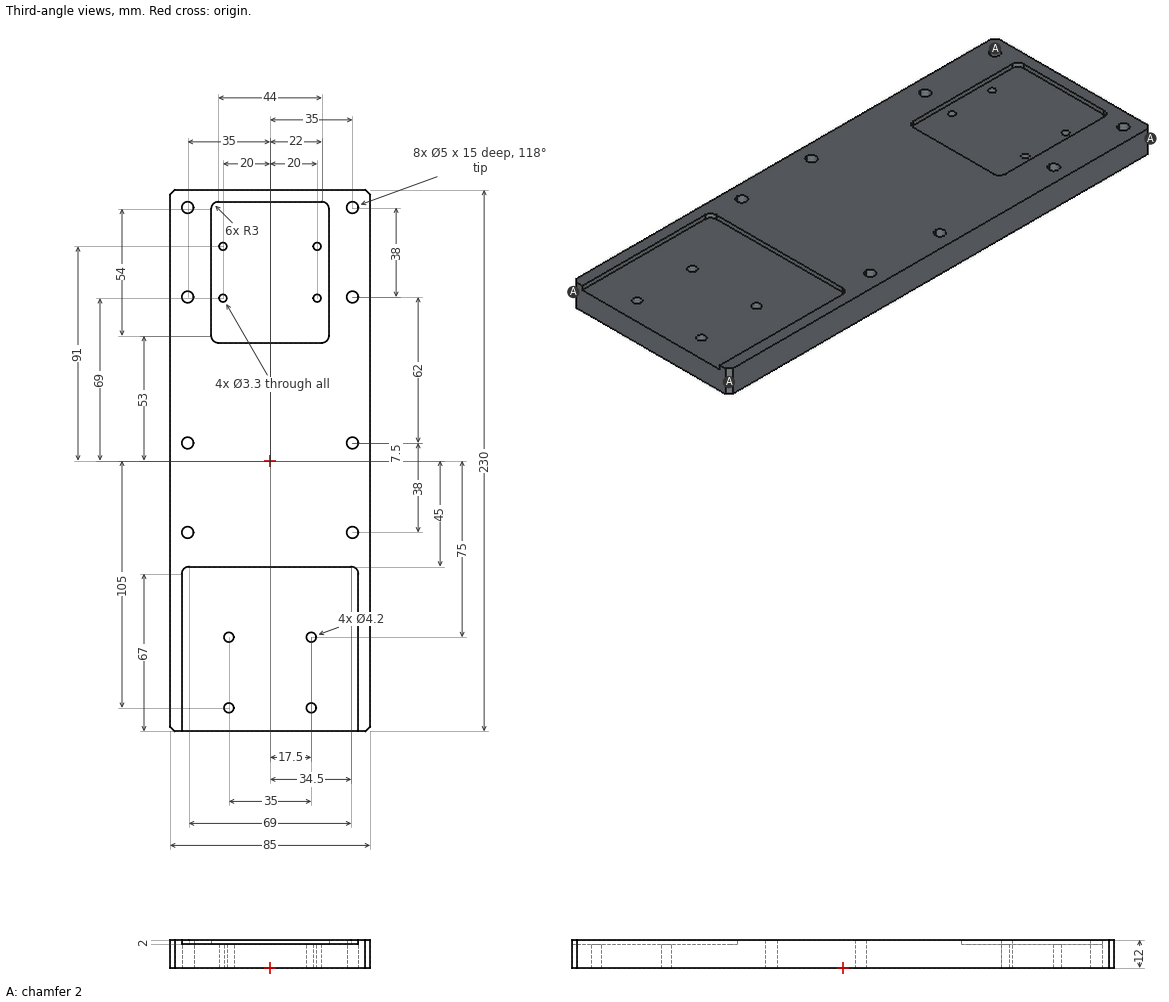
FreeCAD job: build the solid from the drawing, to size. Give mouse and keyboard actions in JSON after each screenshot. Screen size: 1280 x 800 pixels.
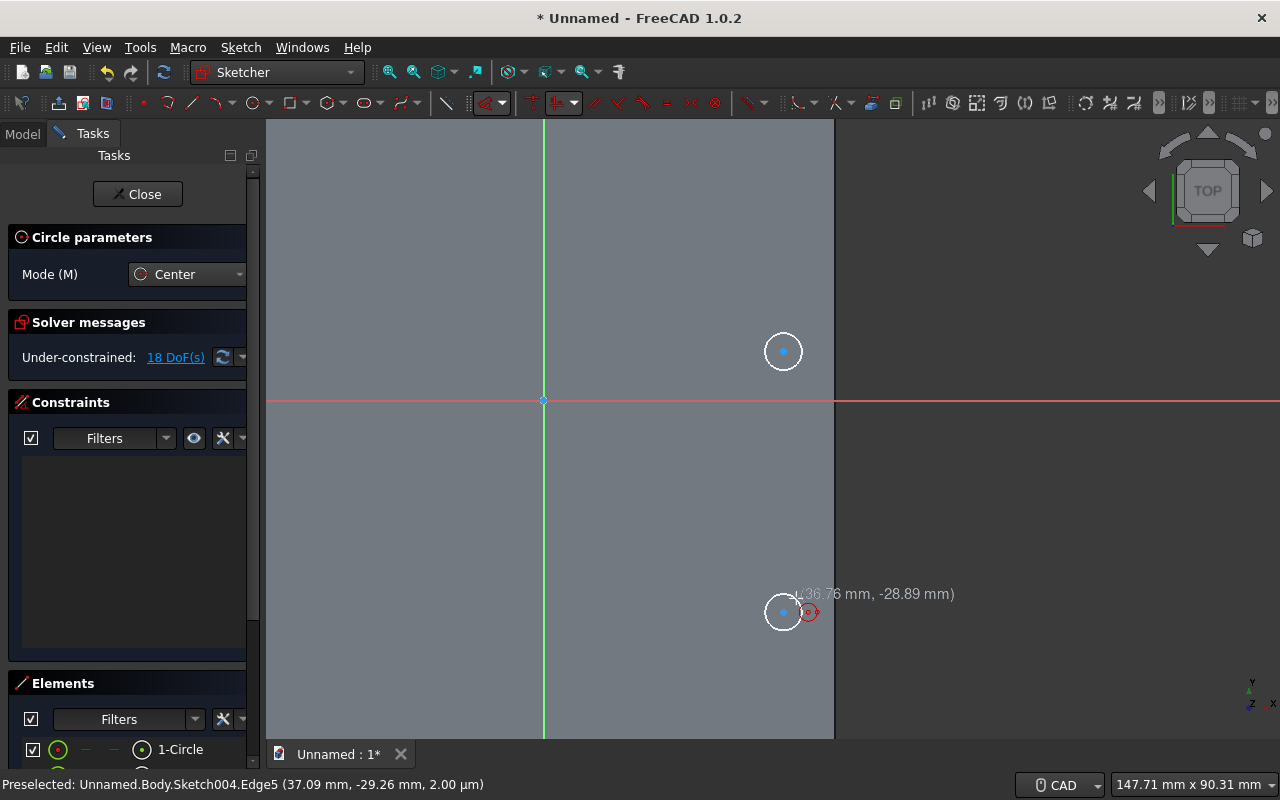
{"action": "scroll", "coordinate": [303, 610], "scroll_direction": "up", "scroll_amount": 2}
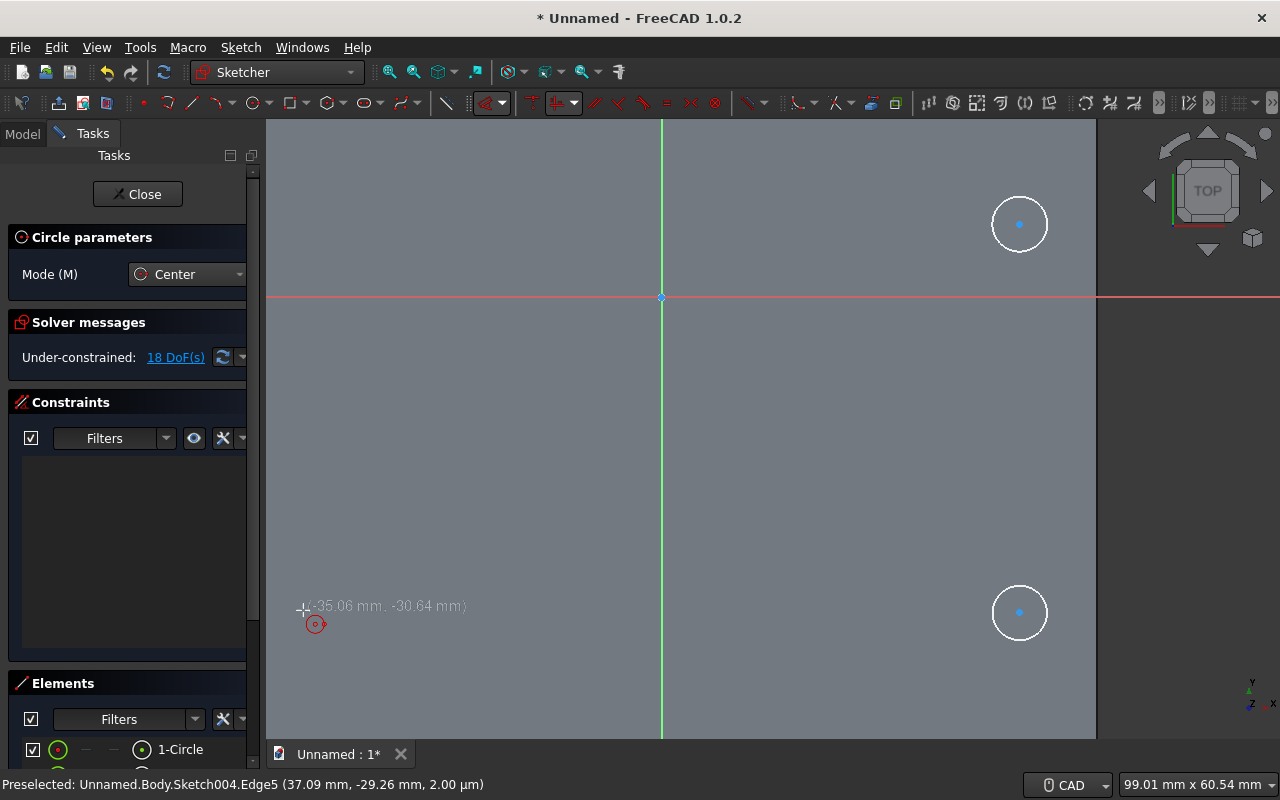
{"action": "scroll", "coordinate": [718, 601], "scroll_direction": "down", "scroll_amount": 7}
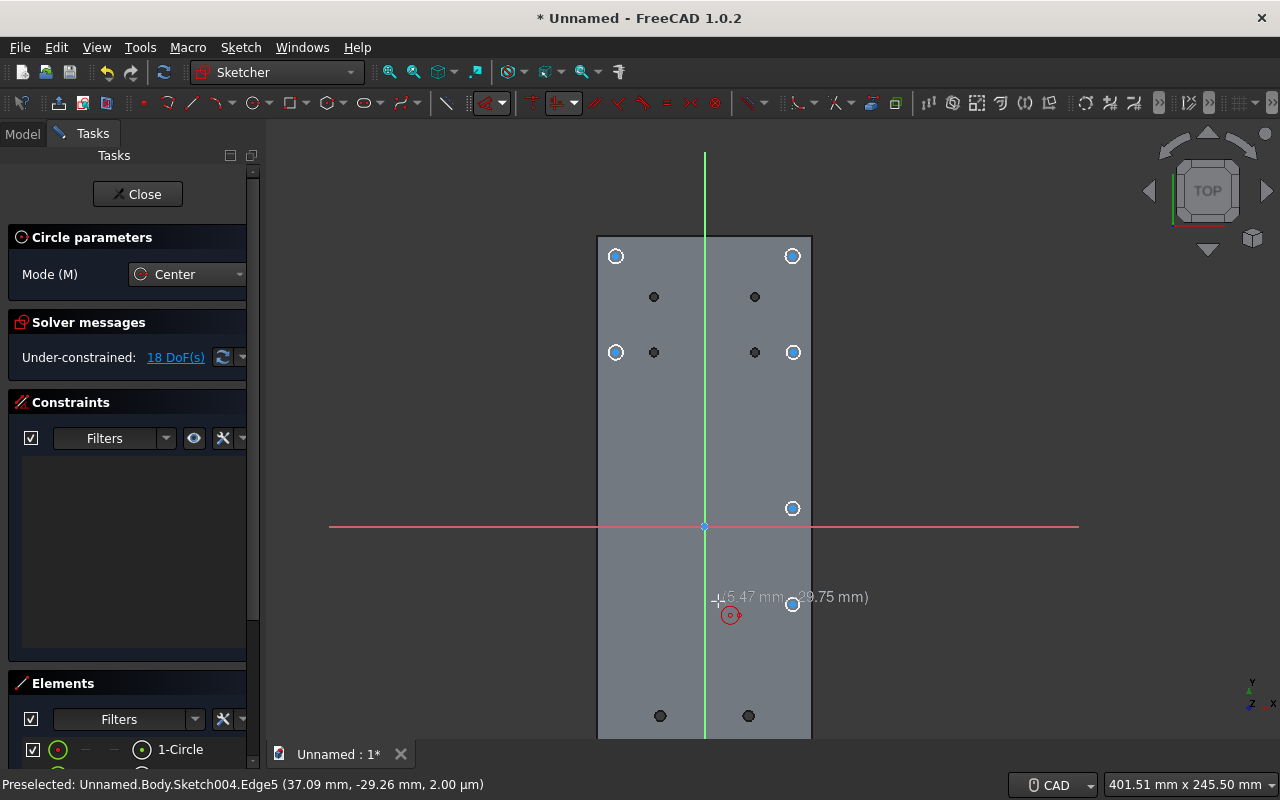
{"action": "left_click", "coordinate": [616, 604]}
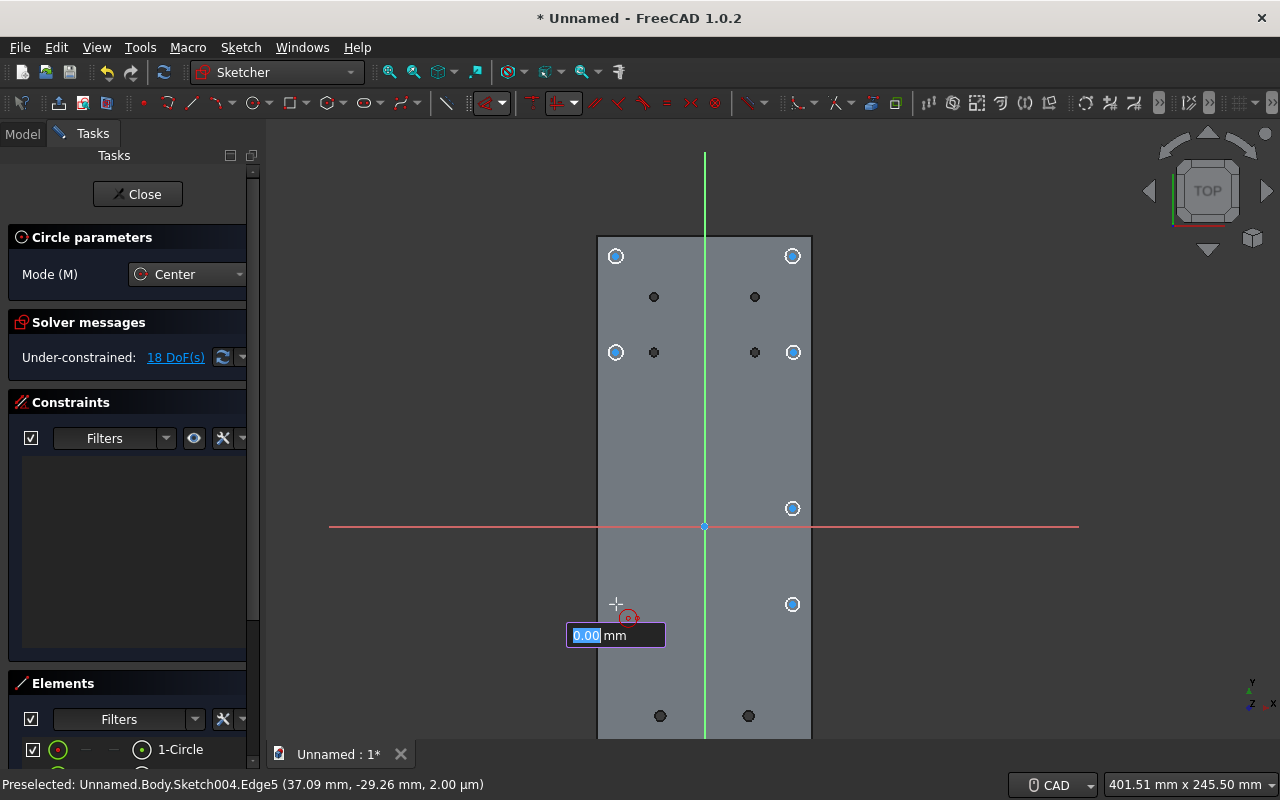
{"action": "scroll", "coordinate": [621, 599], "scroll_direction": "up", "scroll_amount": 5}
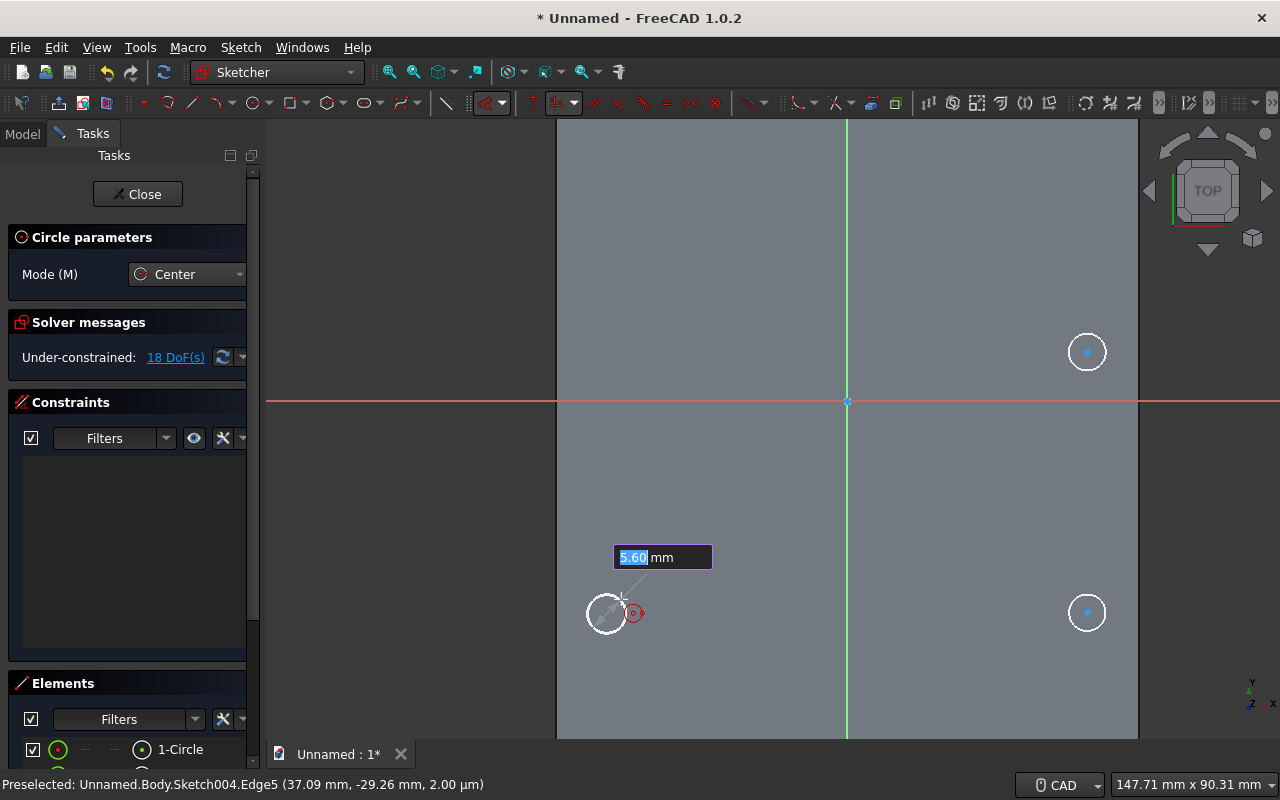
{"action": "left_click", "coordinate": [619, 598]}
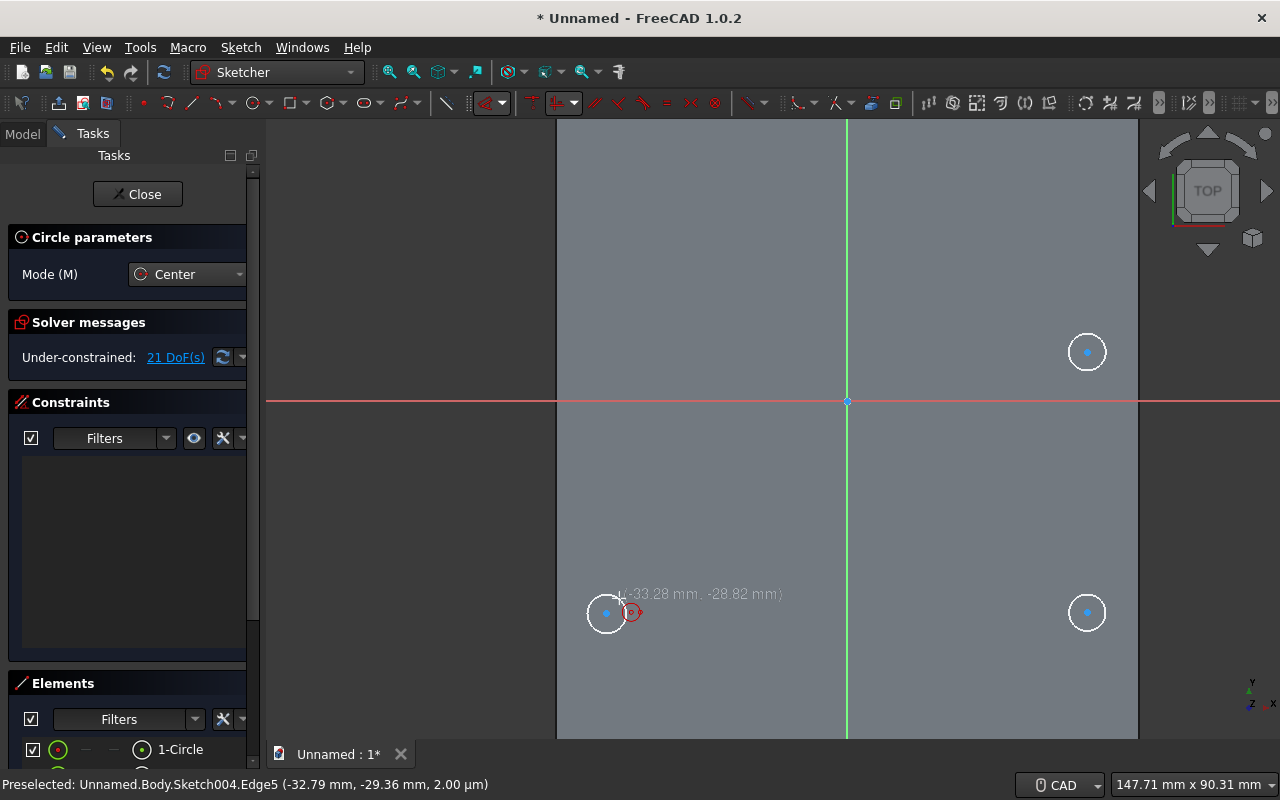
{"action": "scroll", "coordinate": [607, 350], "scroll_direction": "up", "scroll_amount": 2}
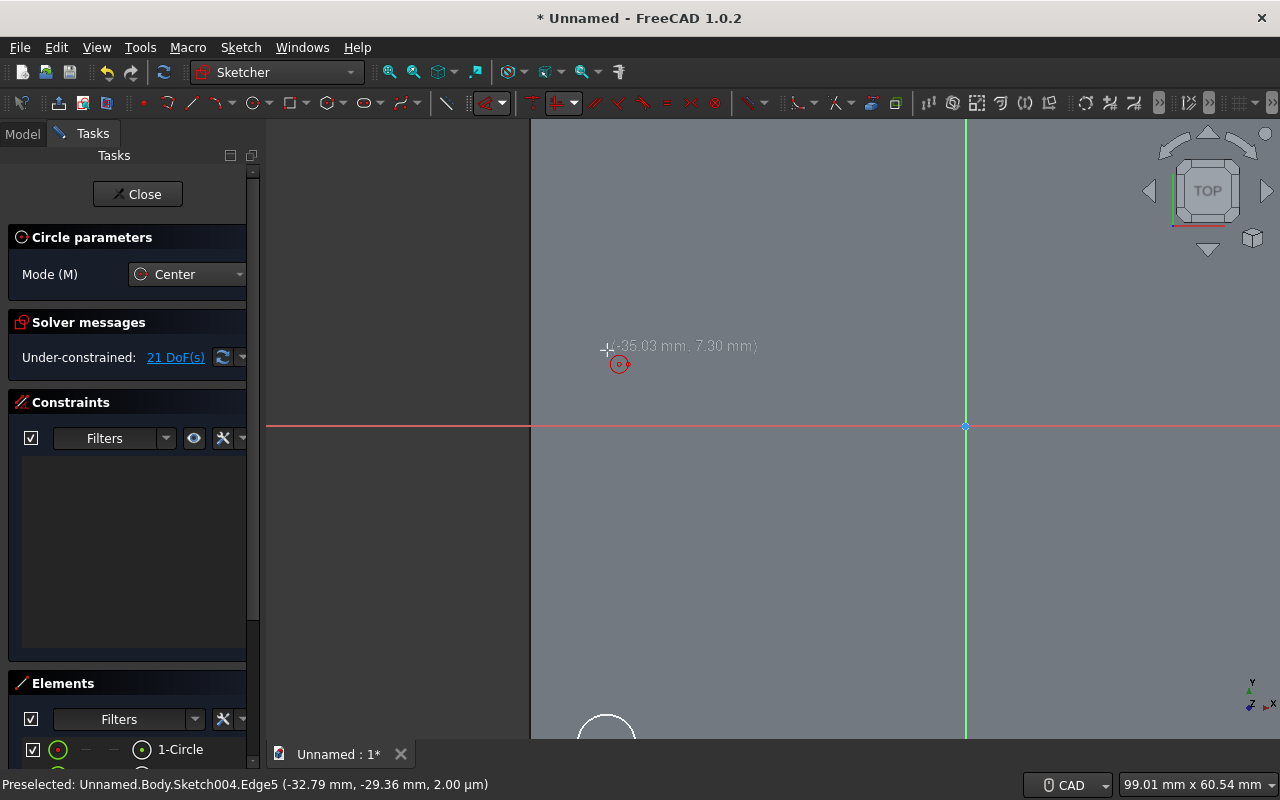
{"action": "scroll", "coordinate": [619, 559], "scroll_direction": "down", "scroll_amount": 7}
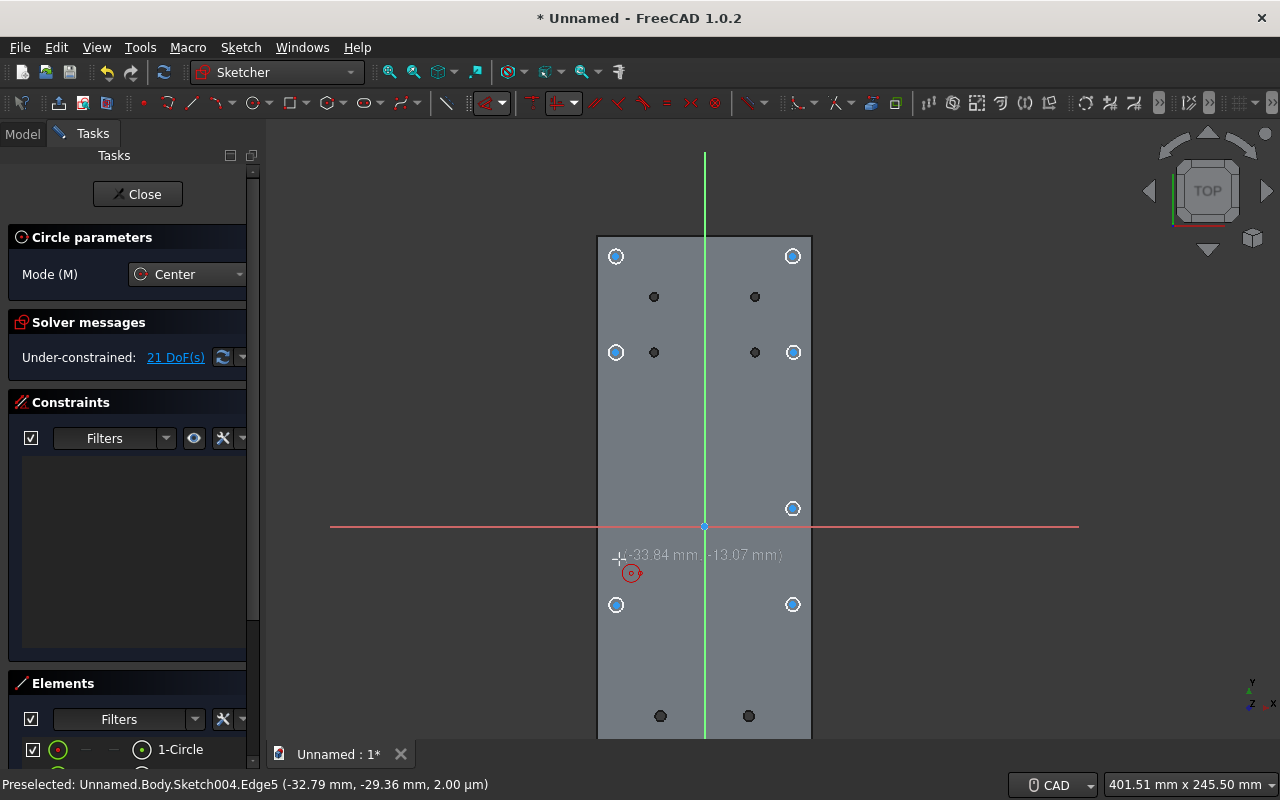
{"action": "left_click", "coordinate": [616, 508]}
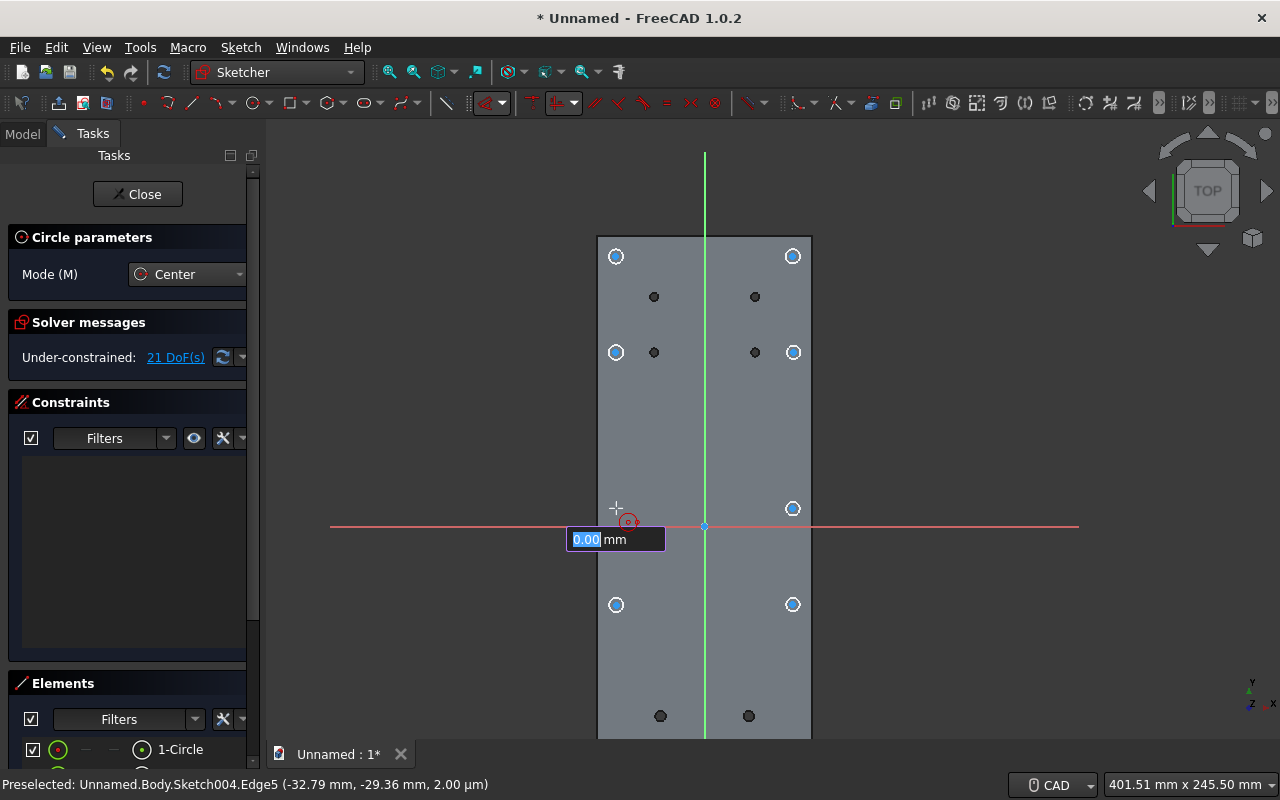
{"action": "scroll", "coordinate": [621, 503], "scroll_direction": "up", "scroll_amount": 5}